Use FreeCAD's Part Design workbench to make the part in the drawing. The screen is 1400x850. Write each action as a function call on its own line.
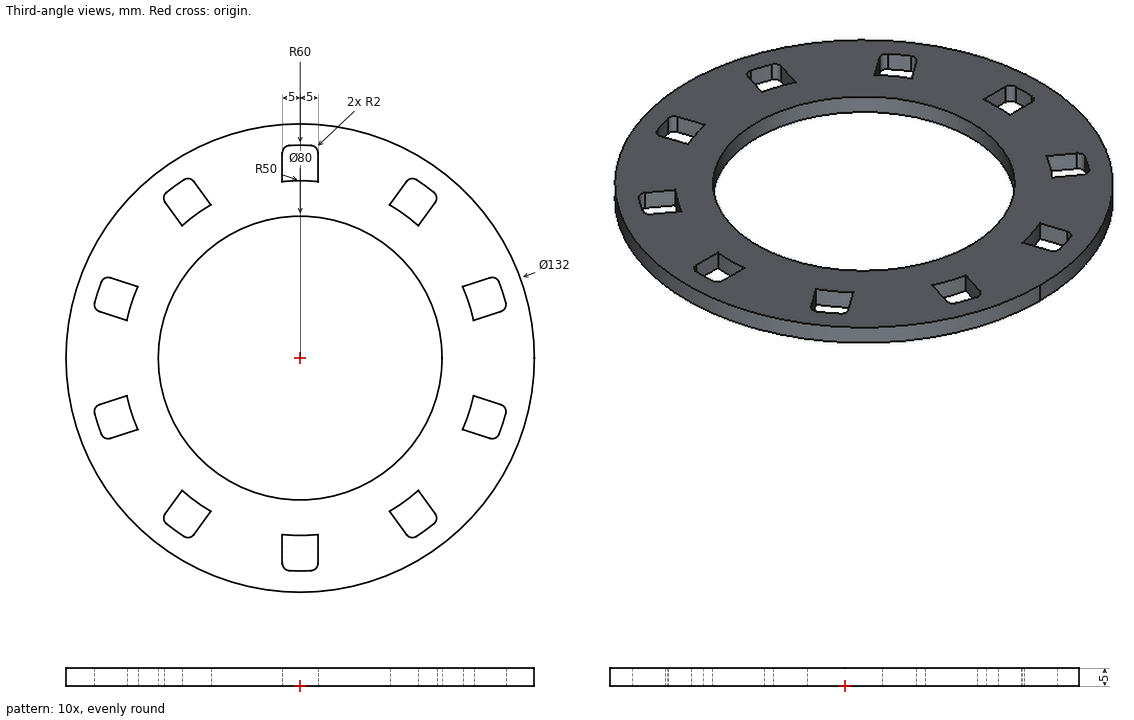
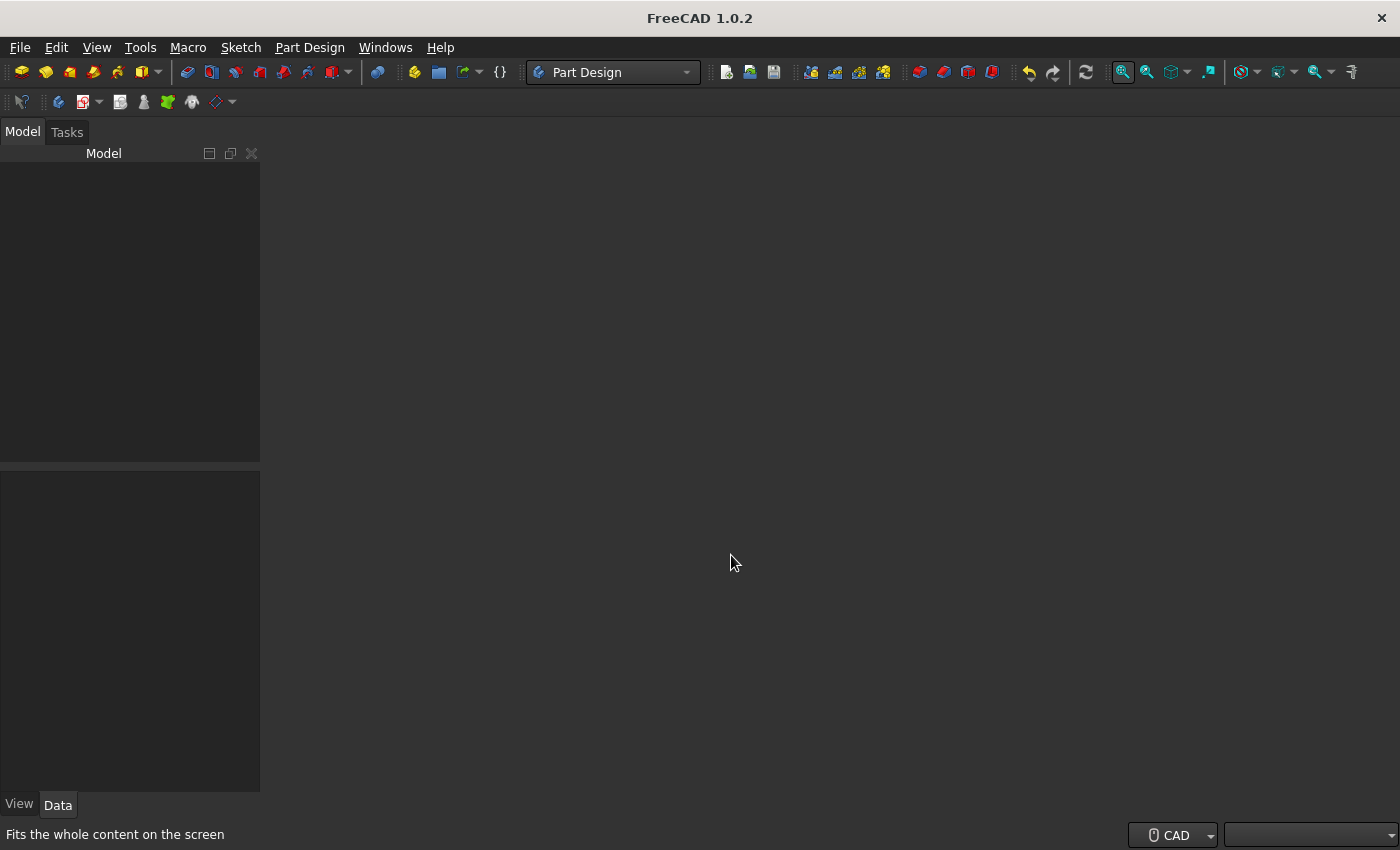
key(ctrl+n)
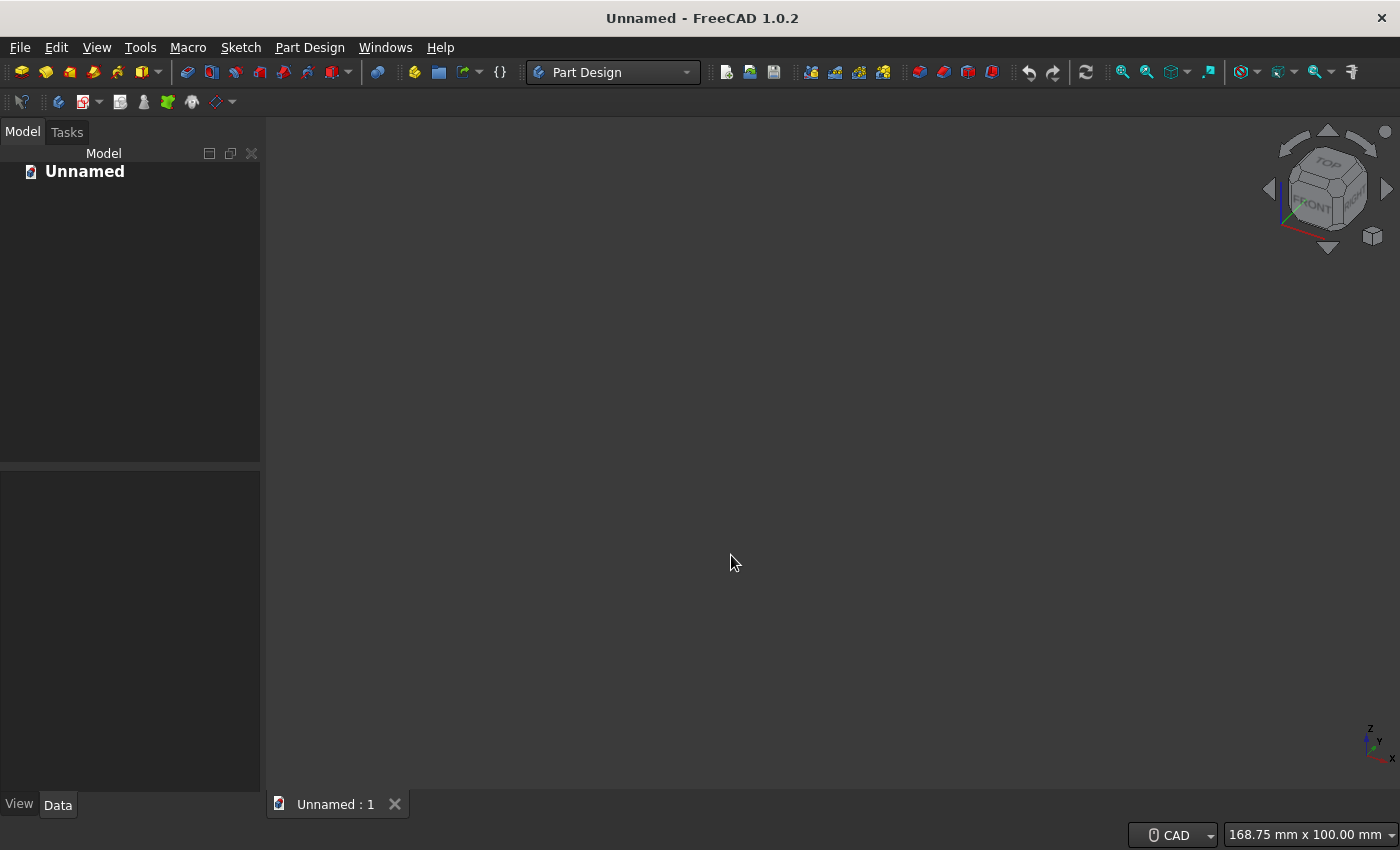
click(84, 102)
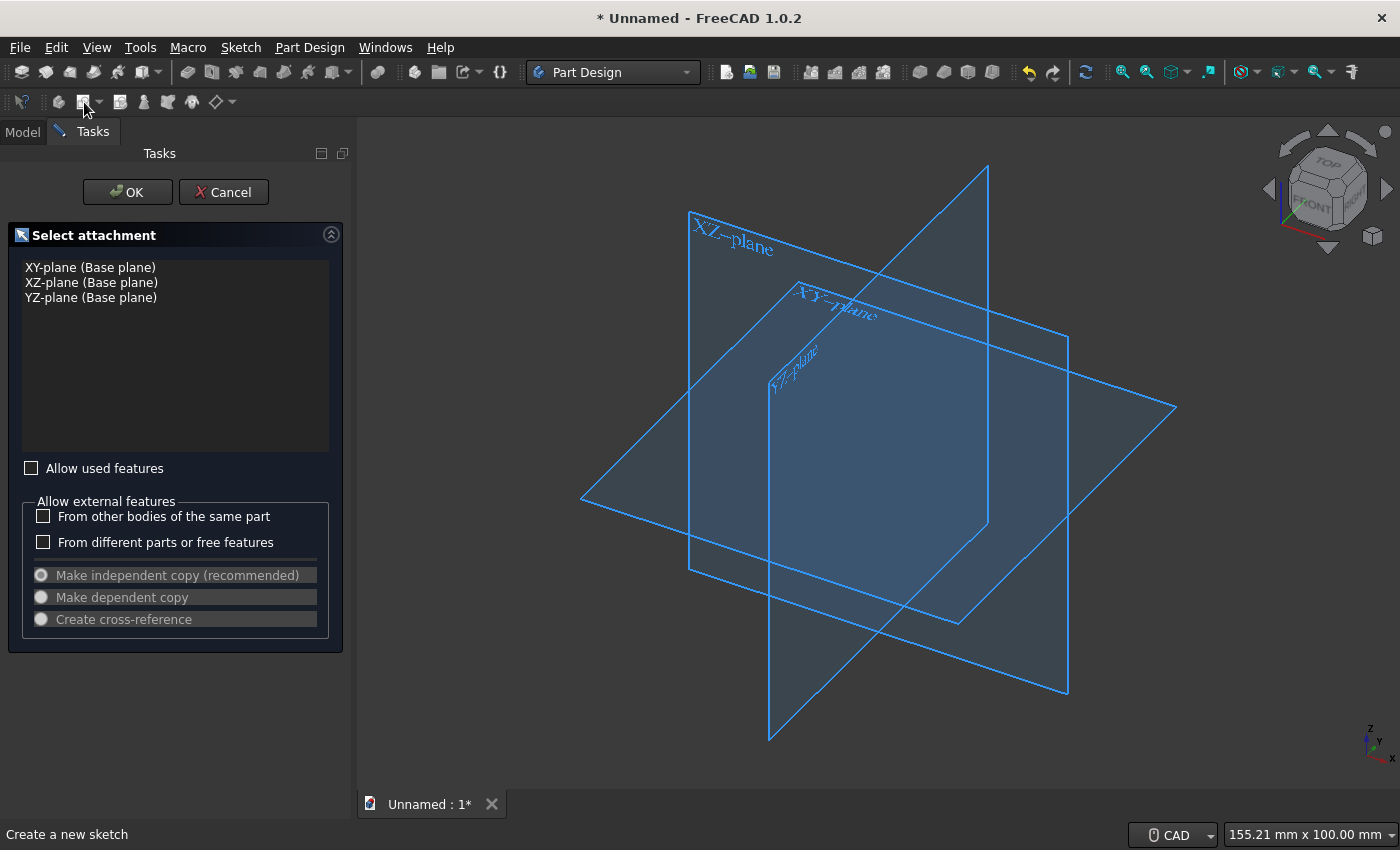
click(82, 268)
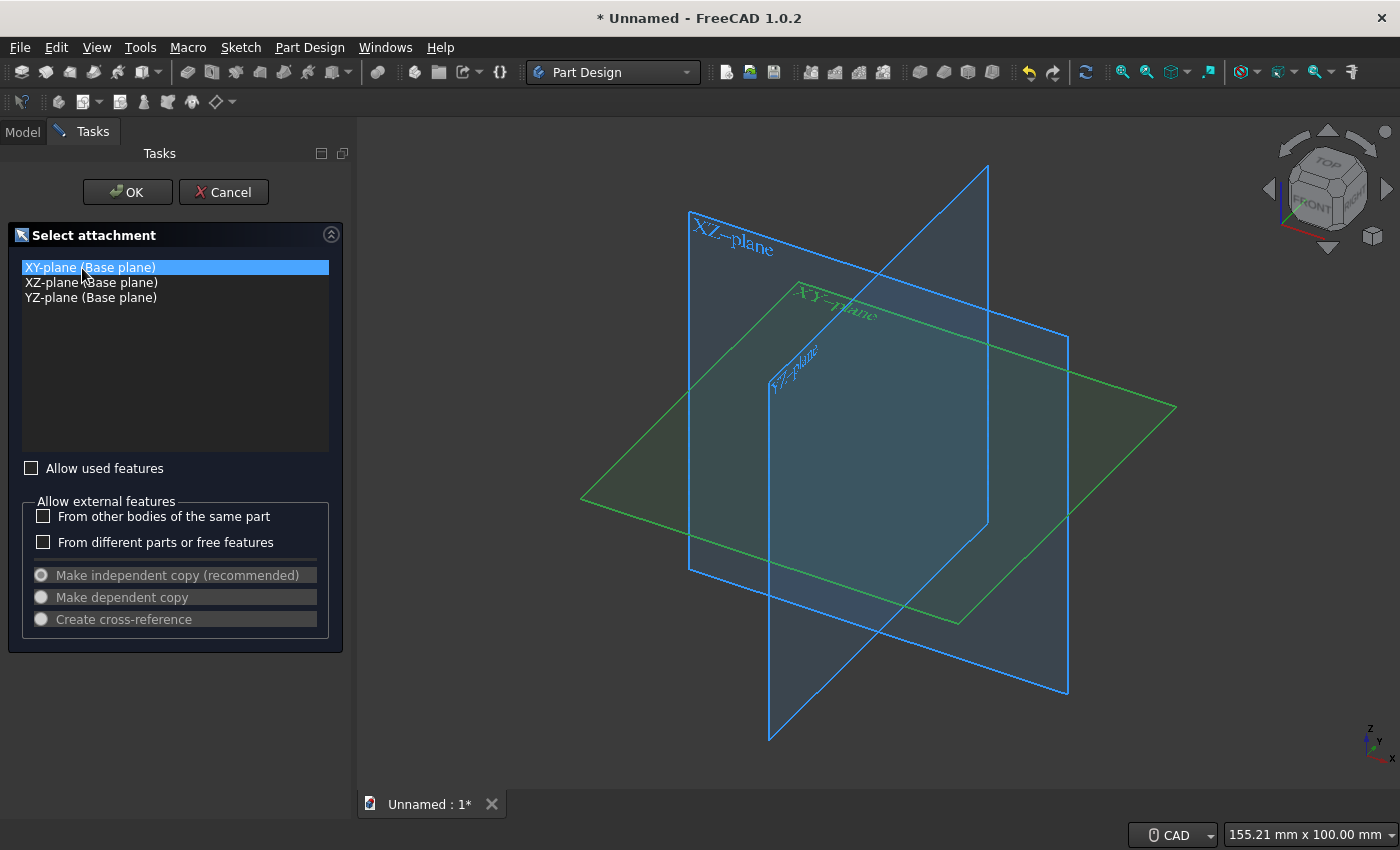
click(128, 192)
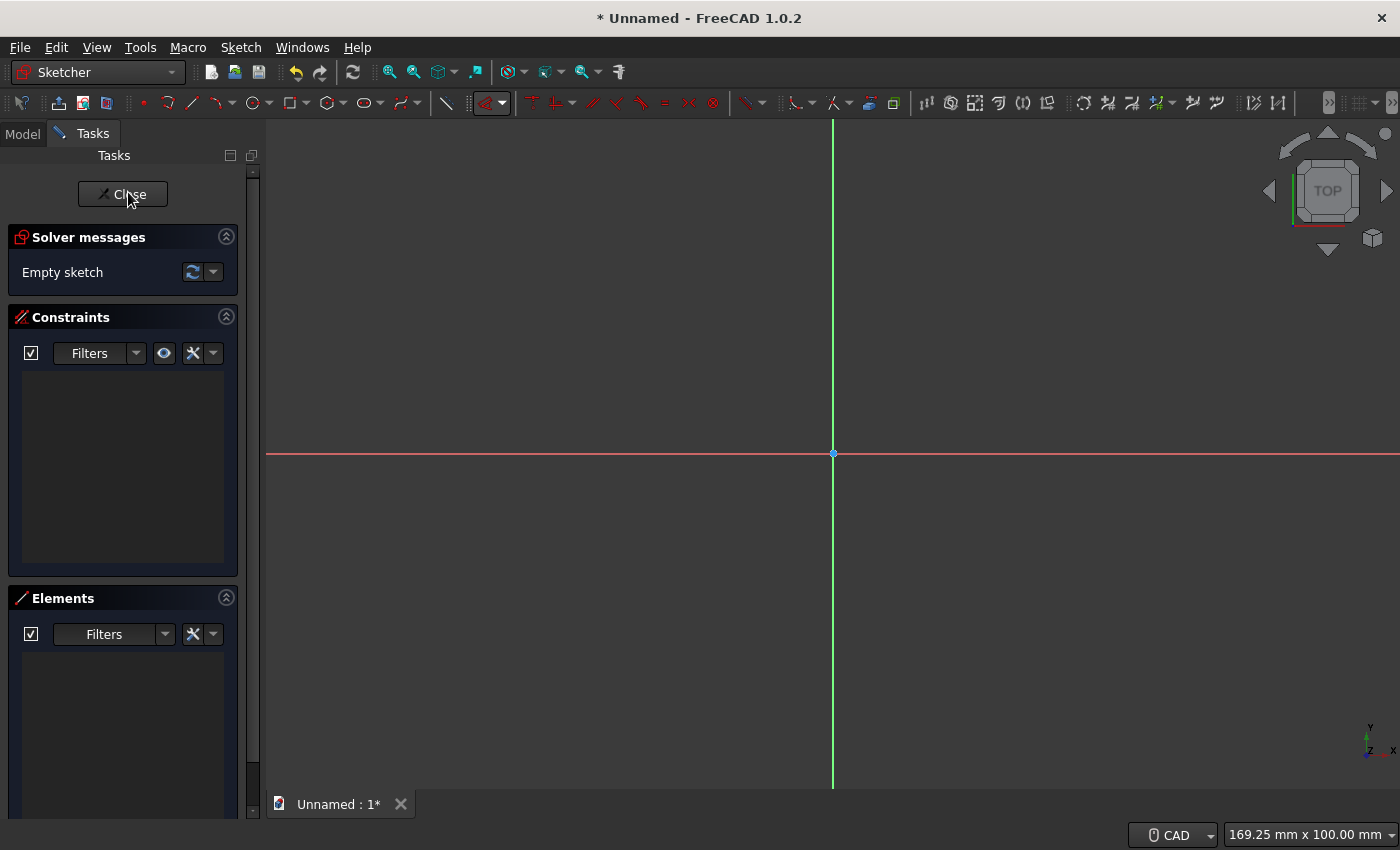
scroll(709, 454, down, 4)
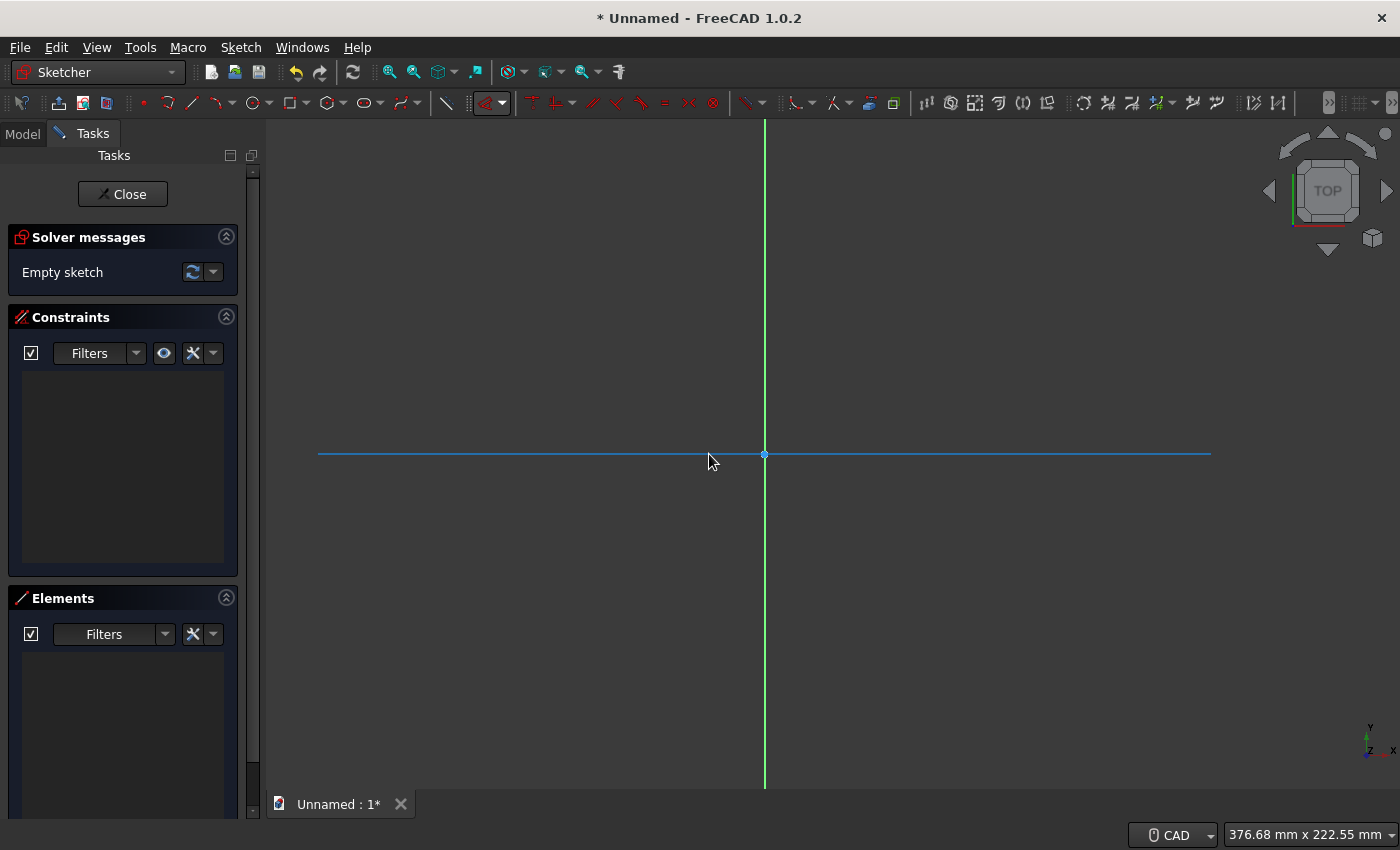
key(g)
key(c)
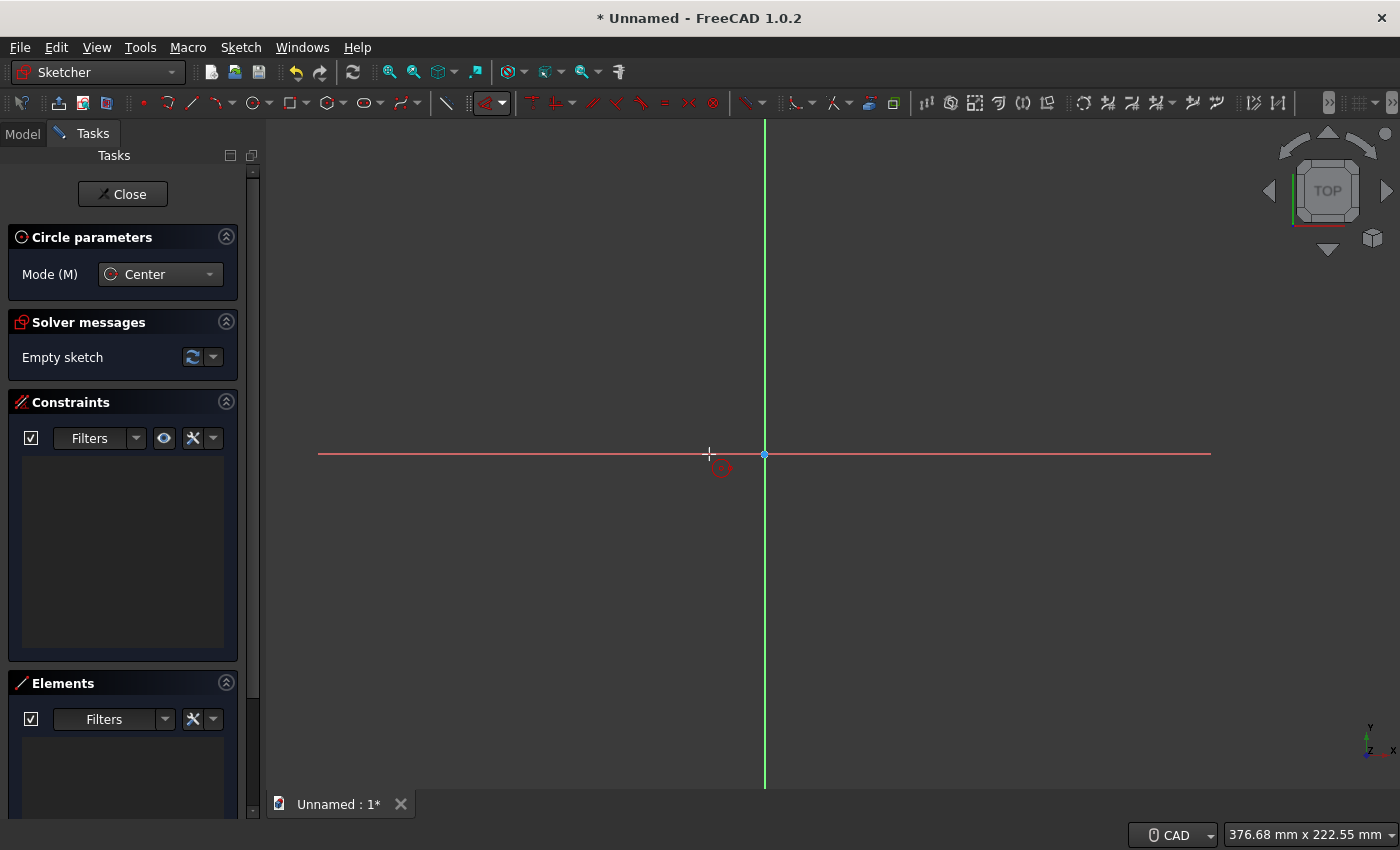
click(765, 454)
move(905, 314)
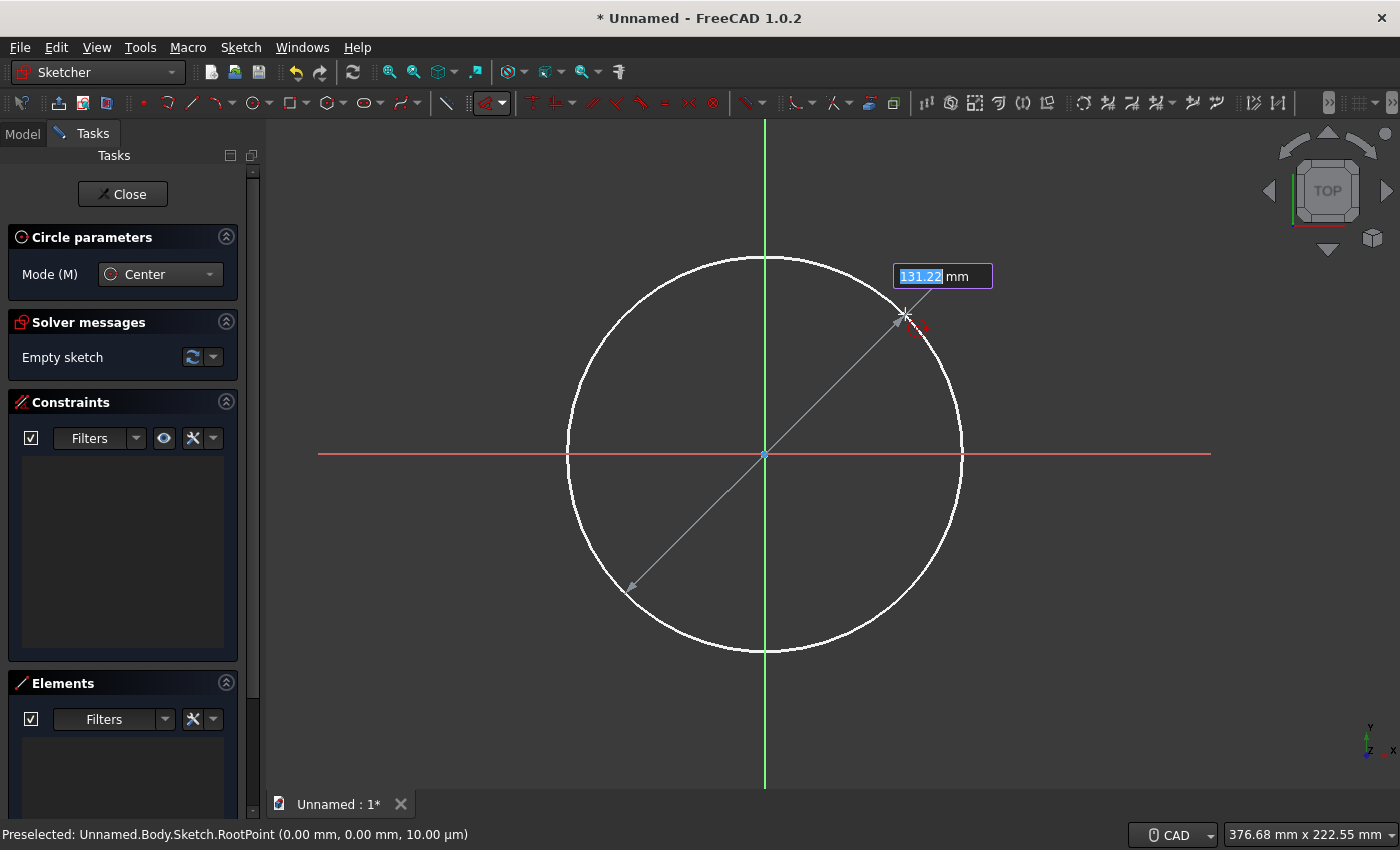
text(132)
key(Return)
key(Escape)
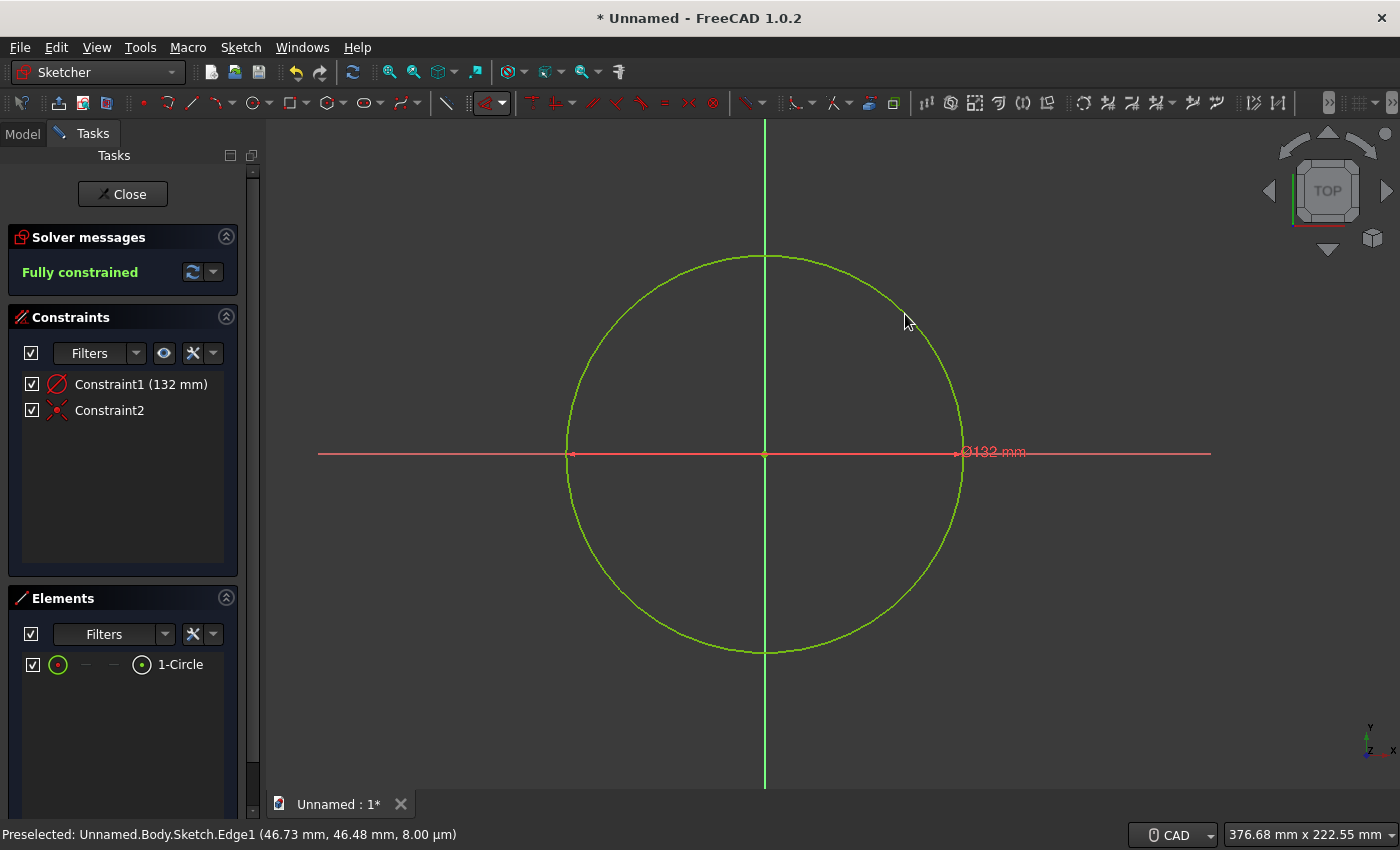
click(123, 194)